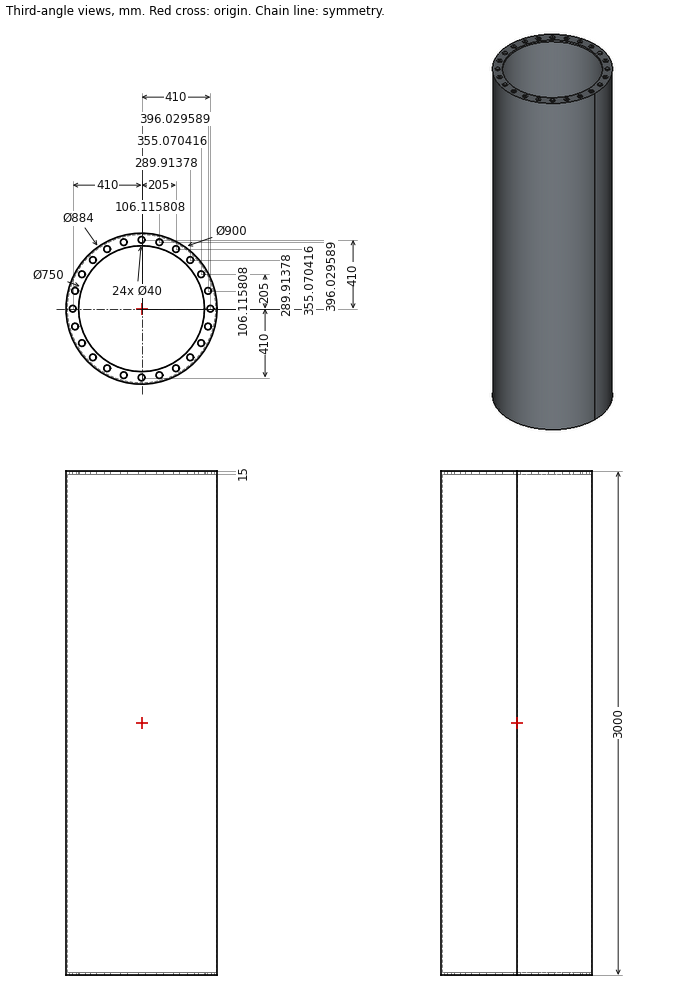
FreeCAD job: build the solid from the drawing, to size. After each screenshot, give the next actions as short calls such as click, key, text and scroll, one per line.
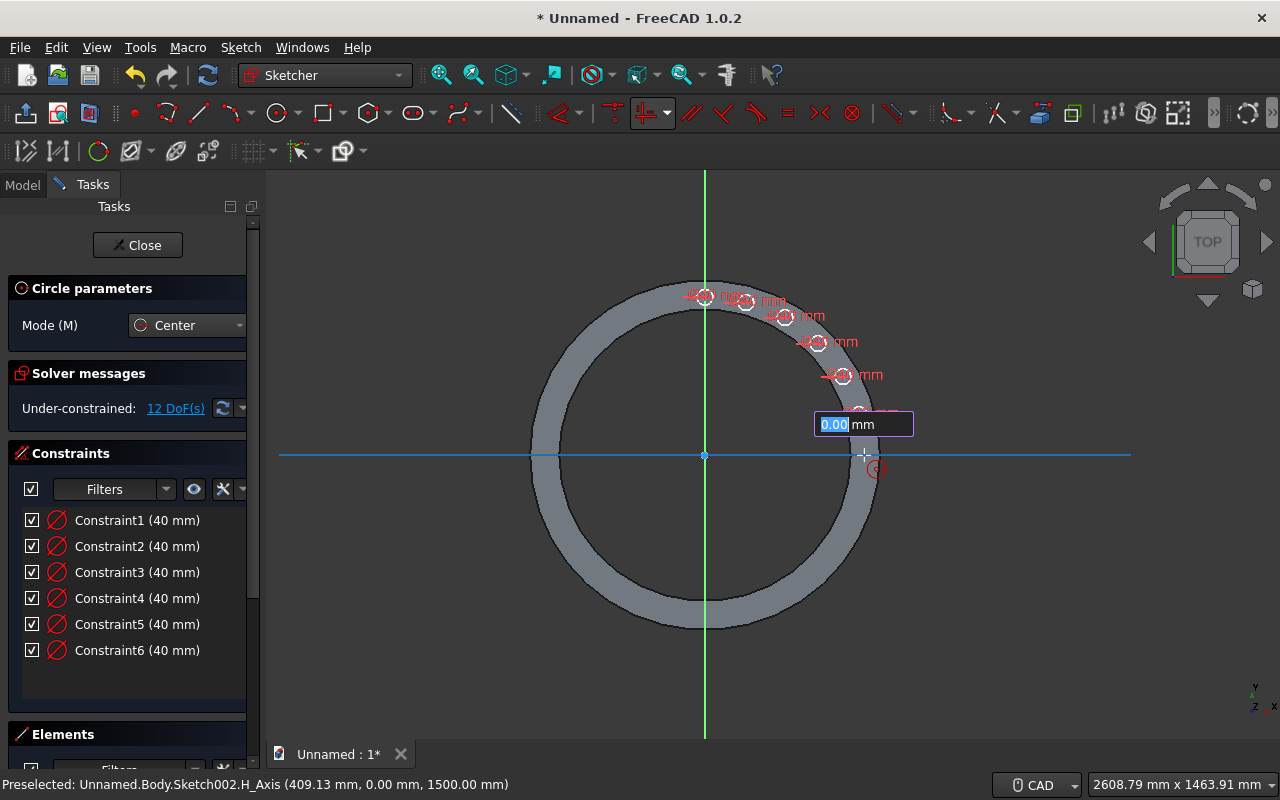
scroll(862, 462, up, 4)
move(861, 462)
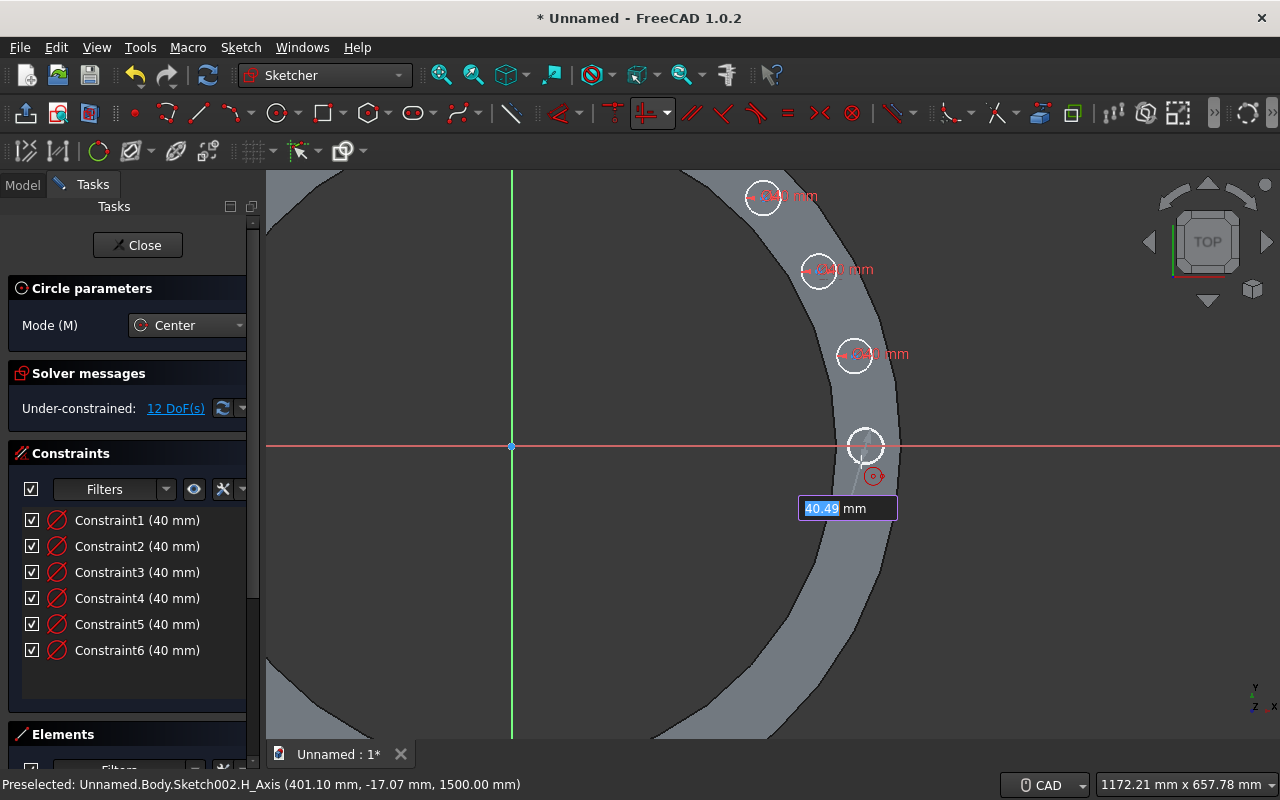
text(40)
key(Return)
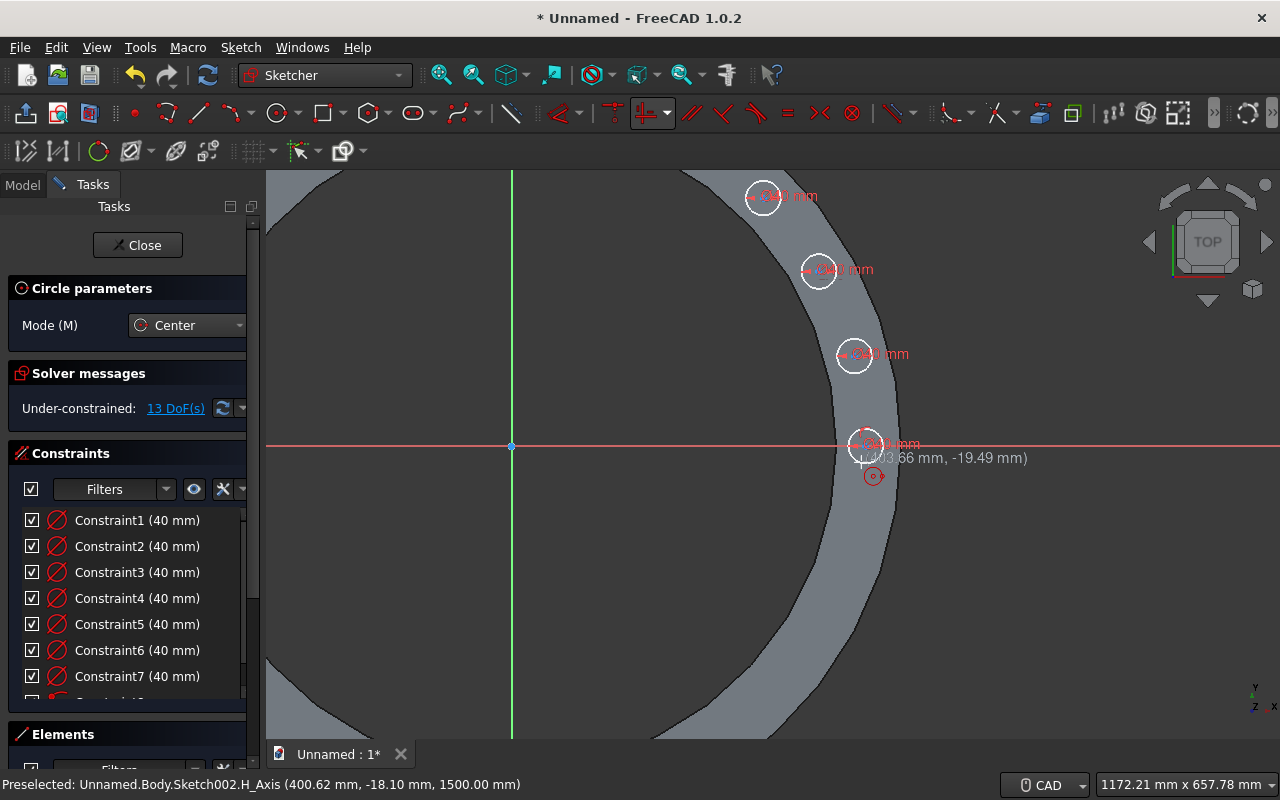
scroll(854, 538, up, 2)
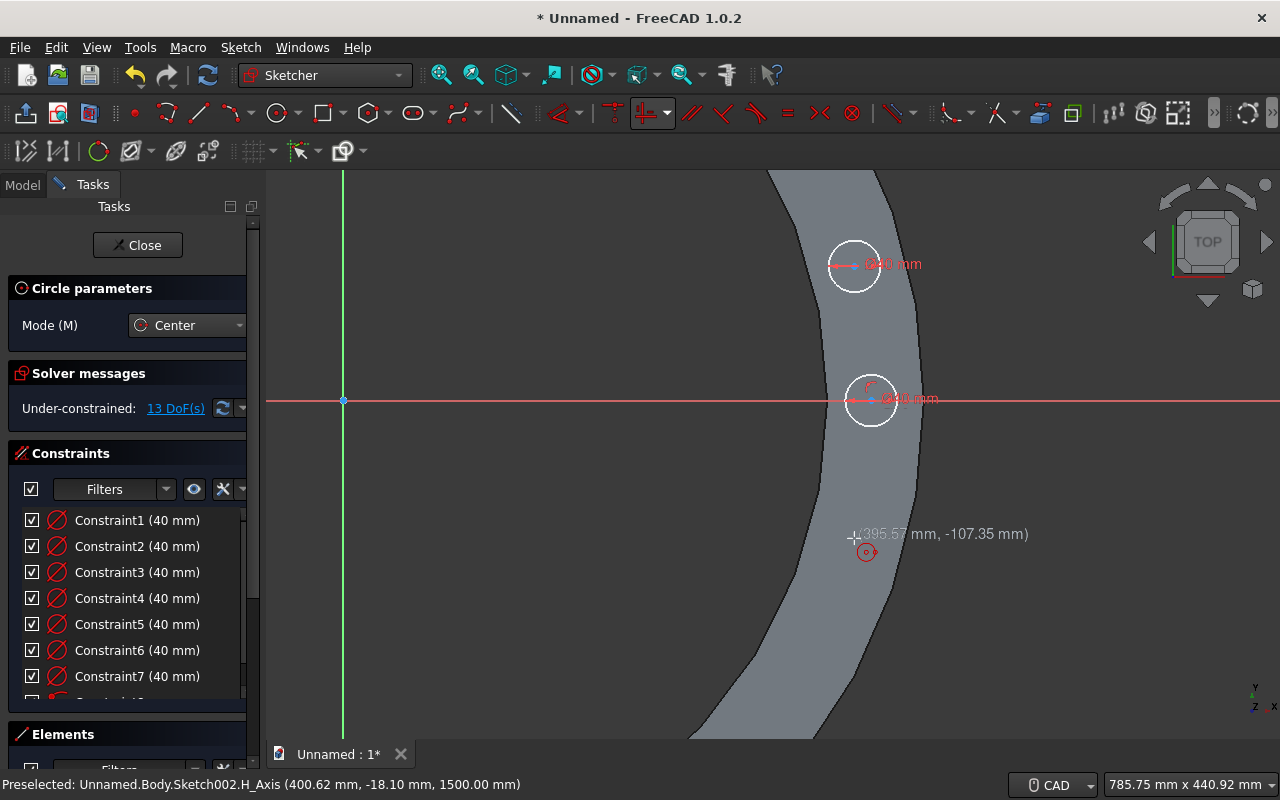
scroll(860, 478, down, 6)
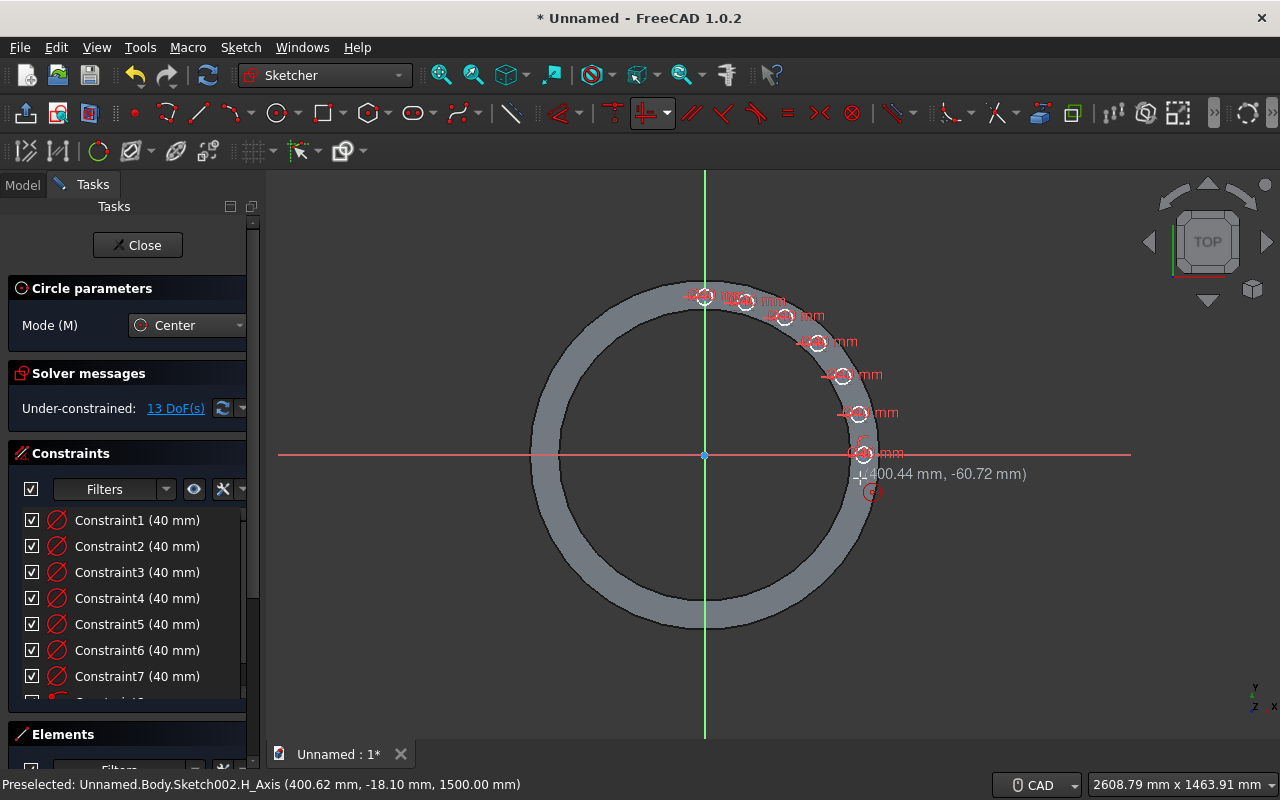
click(859, 496)
move(864, 491)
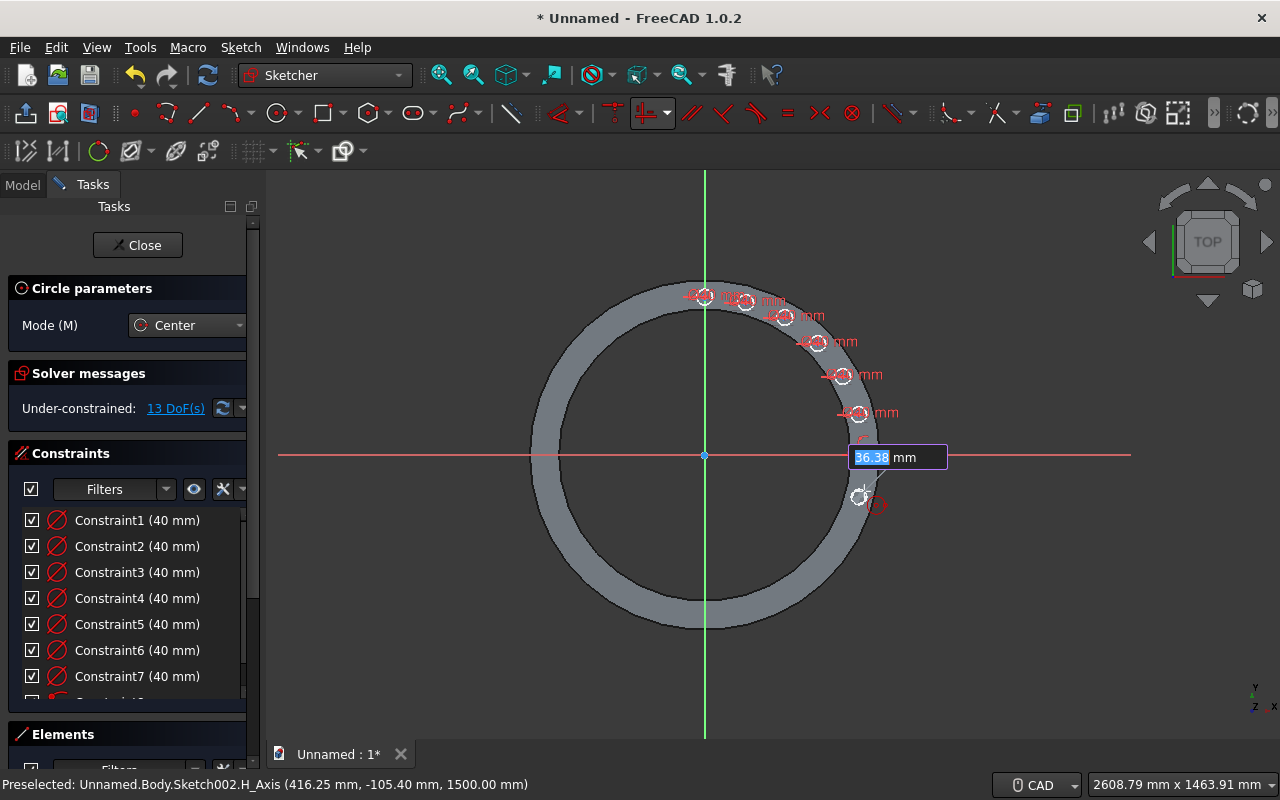
text(40)
key(Return)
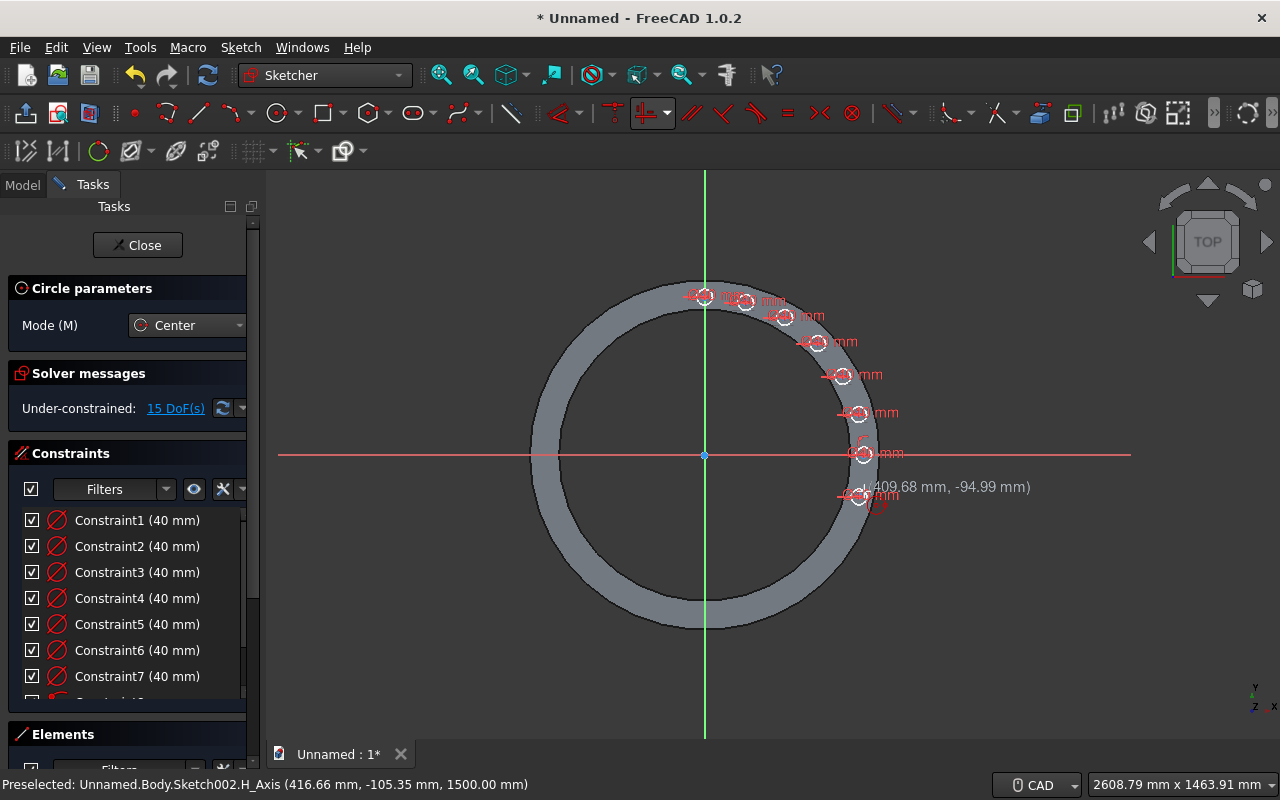
scroll(843, 535, up, 6)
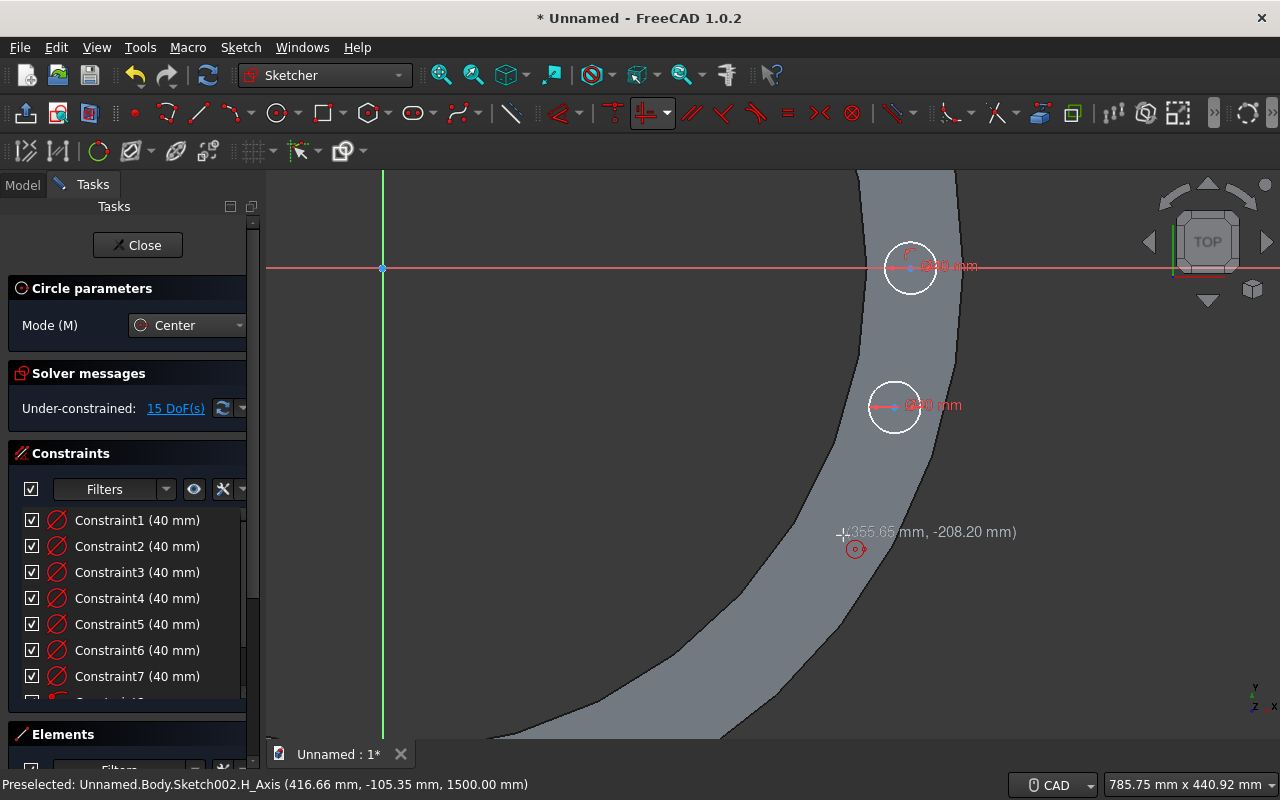
scroll(843, 535, down, 6)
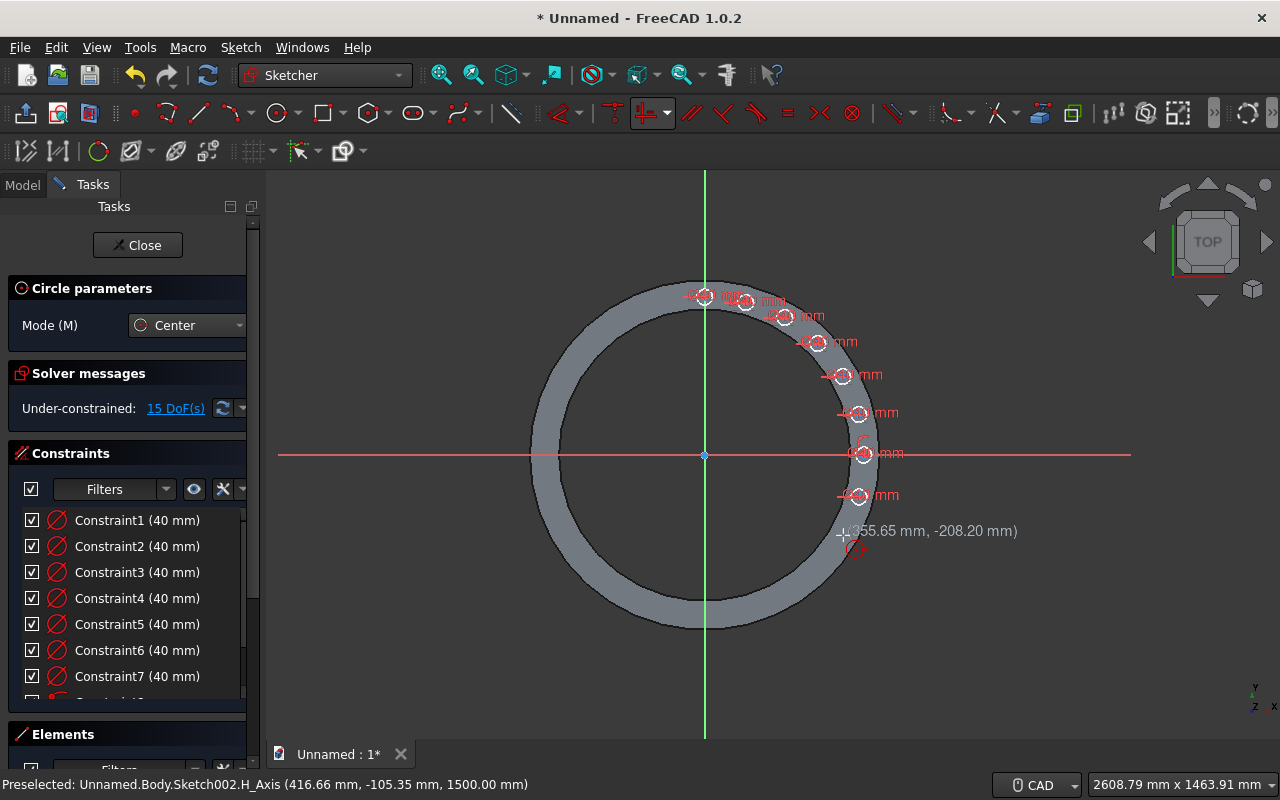
click(843, 535)
move(848, 529)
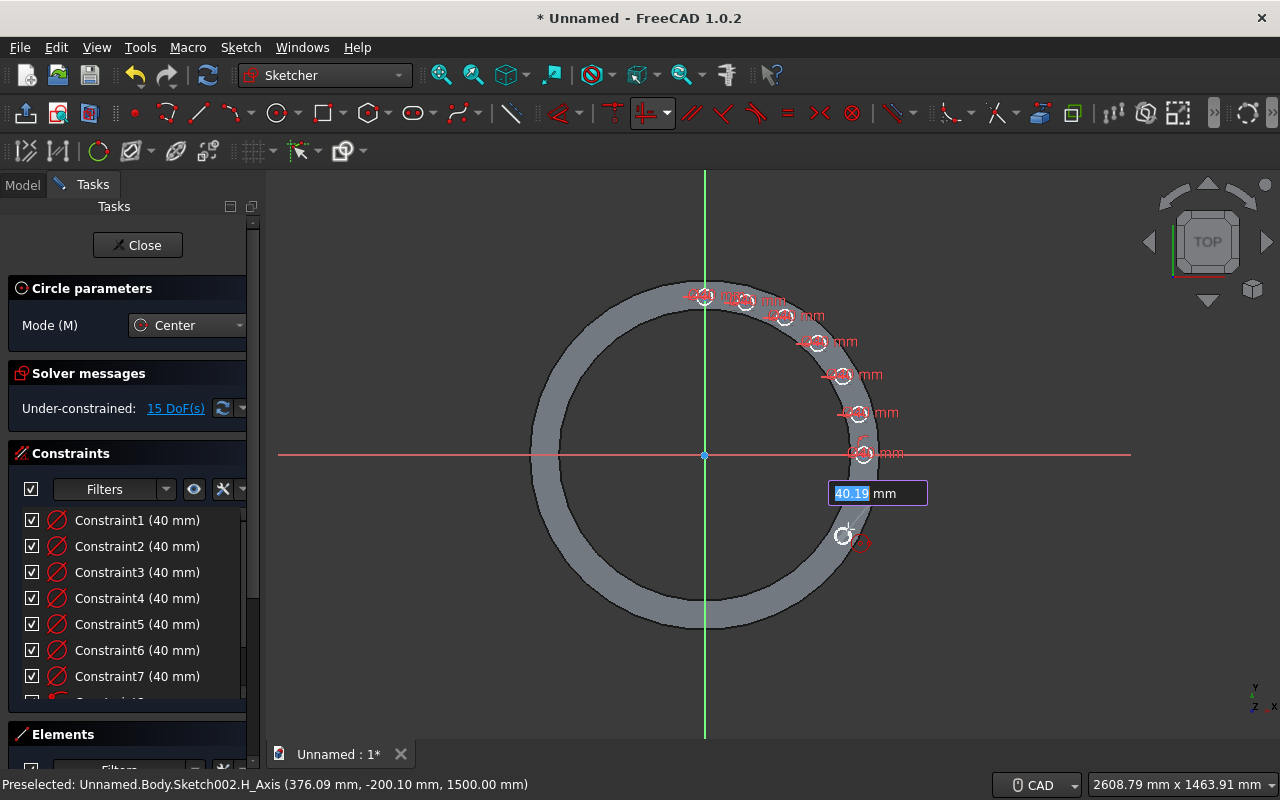
text(40)
key(Return)